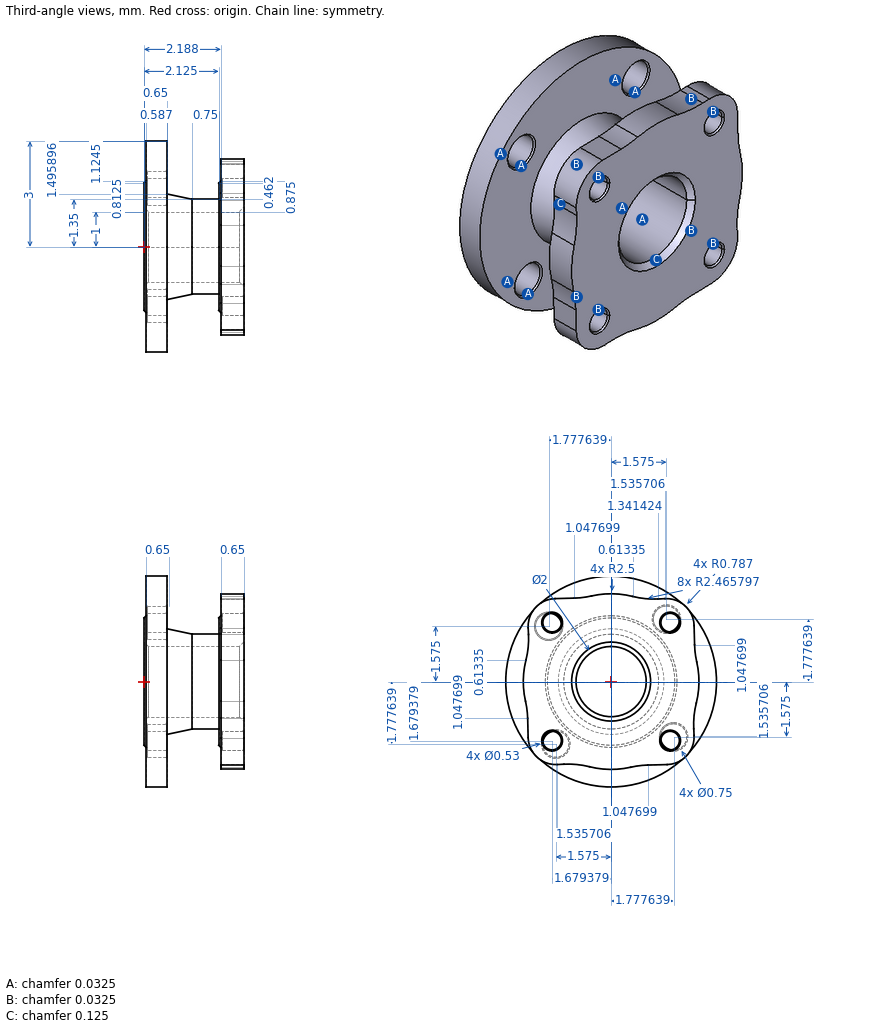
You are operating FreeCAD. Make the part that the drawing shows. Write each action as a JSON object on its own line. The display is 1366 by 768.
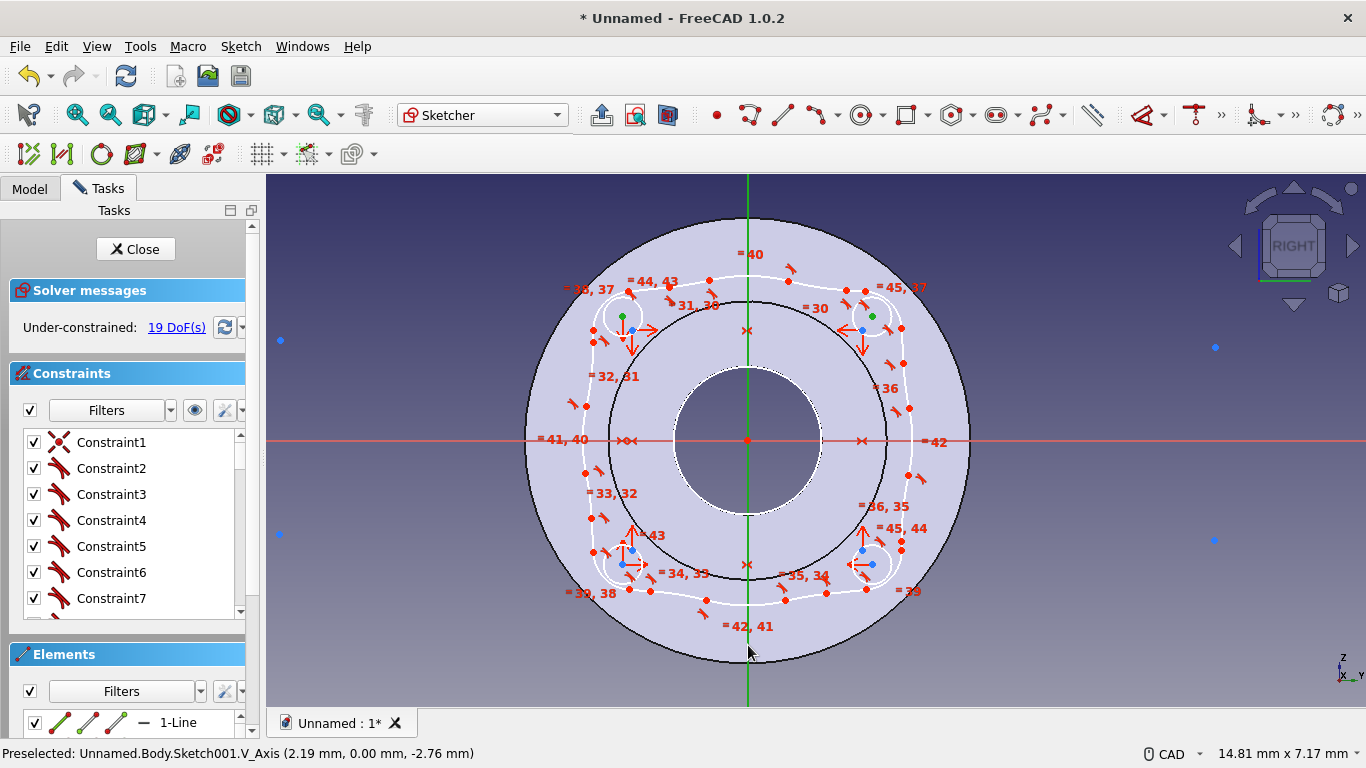
{"action": "key", "text": "s"}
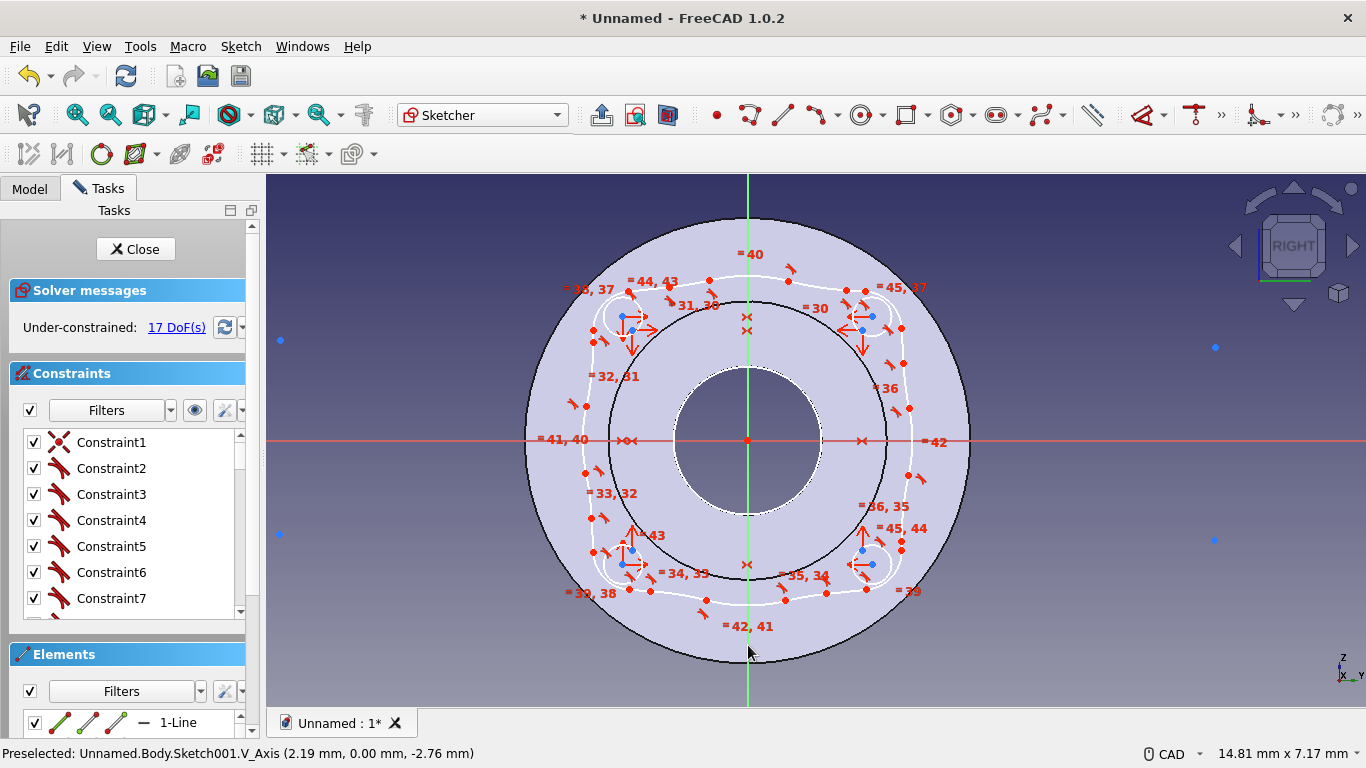
{"action": "left_click", "coordinate": [1142, 116]}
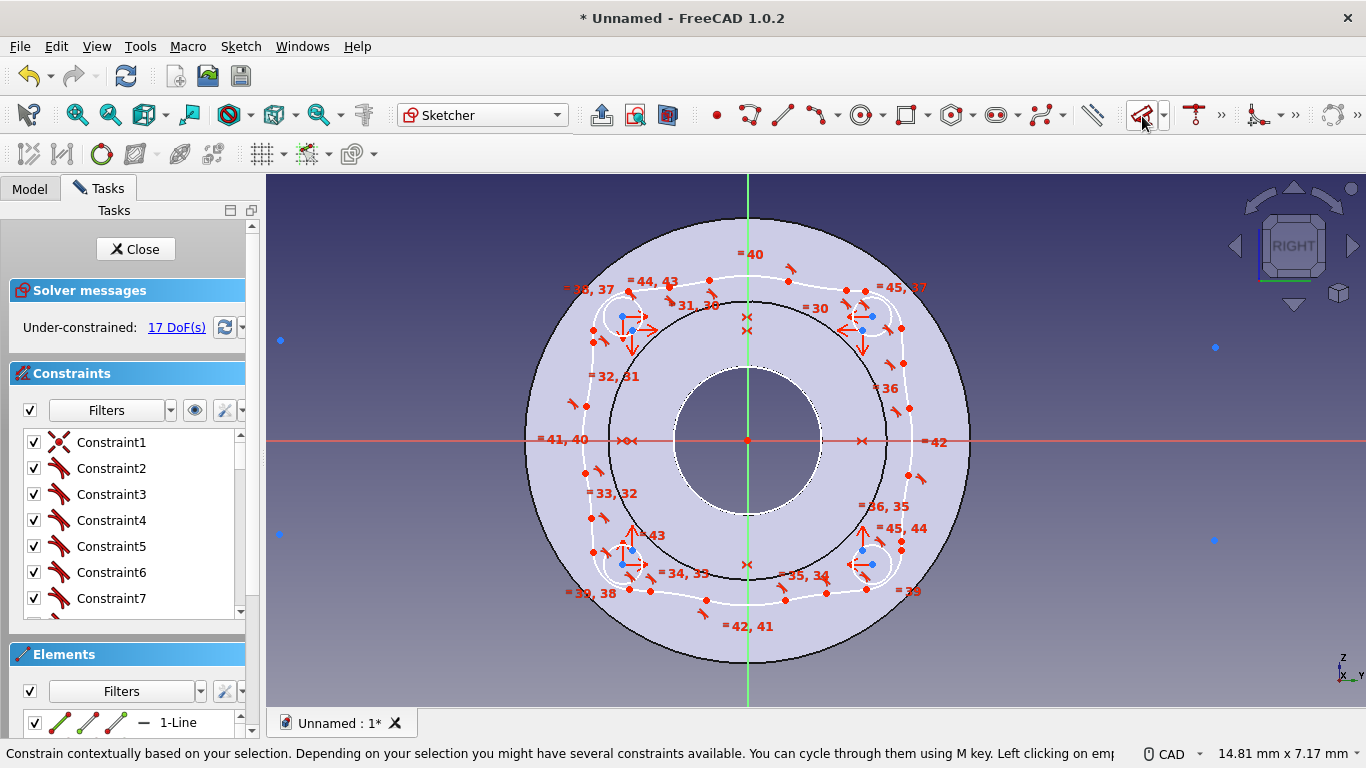
{"action": "scroll", "coordinate": [899, 317], "scroll_direction": "up", "scroll_amount": 3}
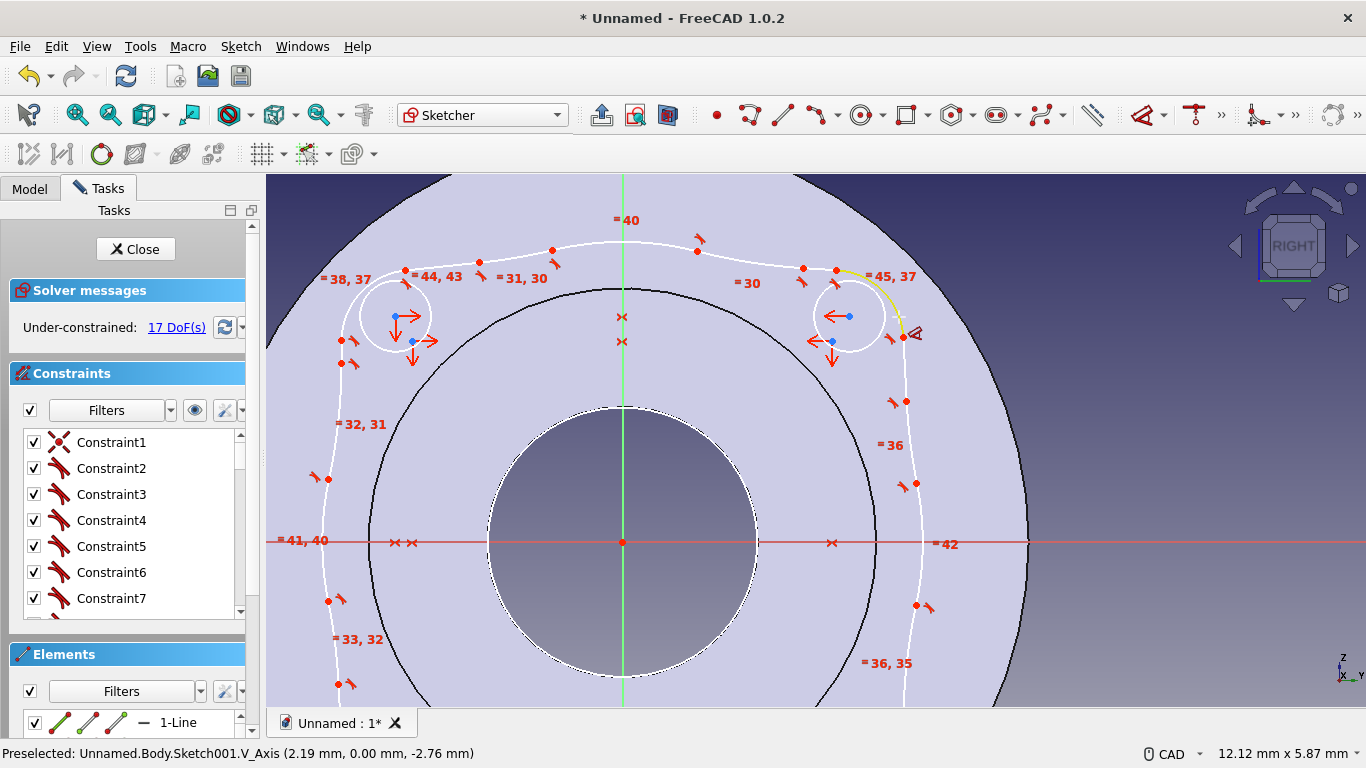
{"action": "left_click", "coordinate": [899, 317]}
{"action": "left_click", "coordinate": [929, 306]}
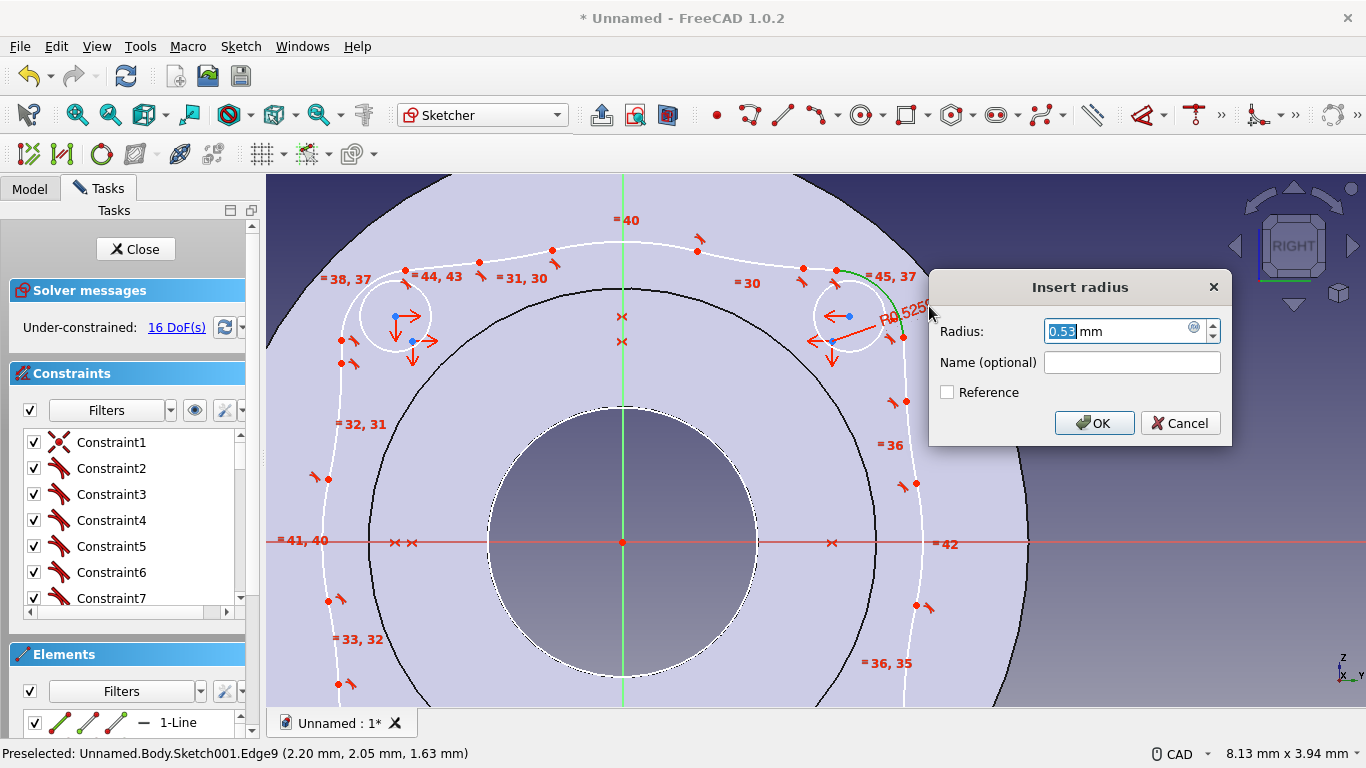
{"action": "type", "text": "0.787"}
{"action": "key", "text": "Return"}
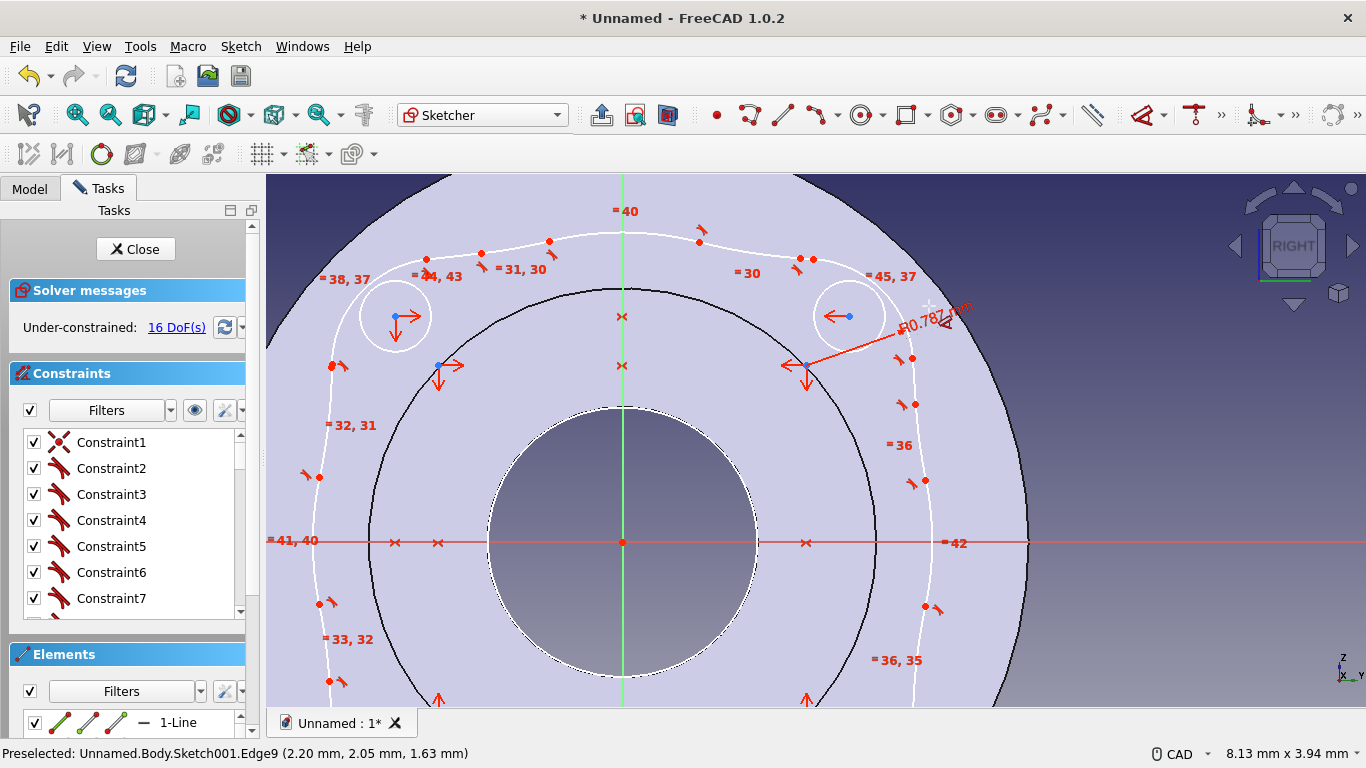
{"action": "left_click", "coordinate": [729, 249]}
{"action": "left_click", "coordinate": [723, 280]}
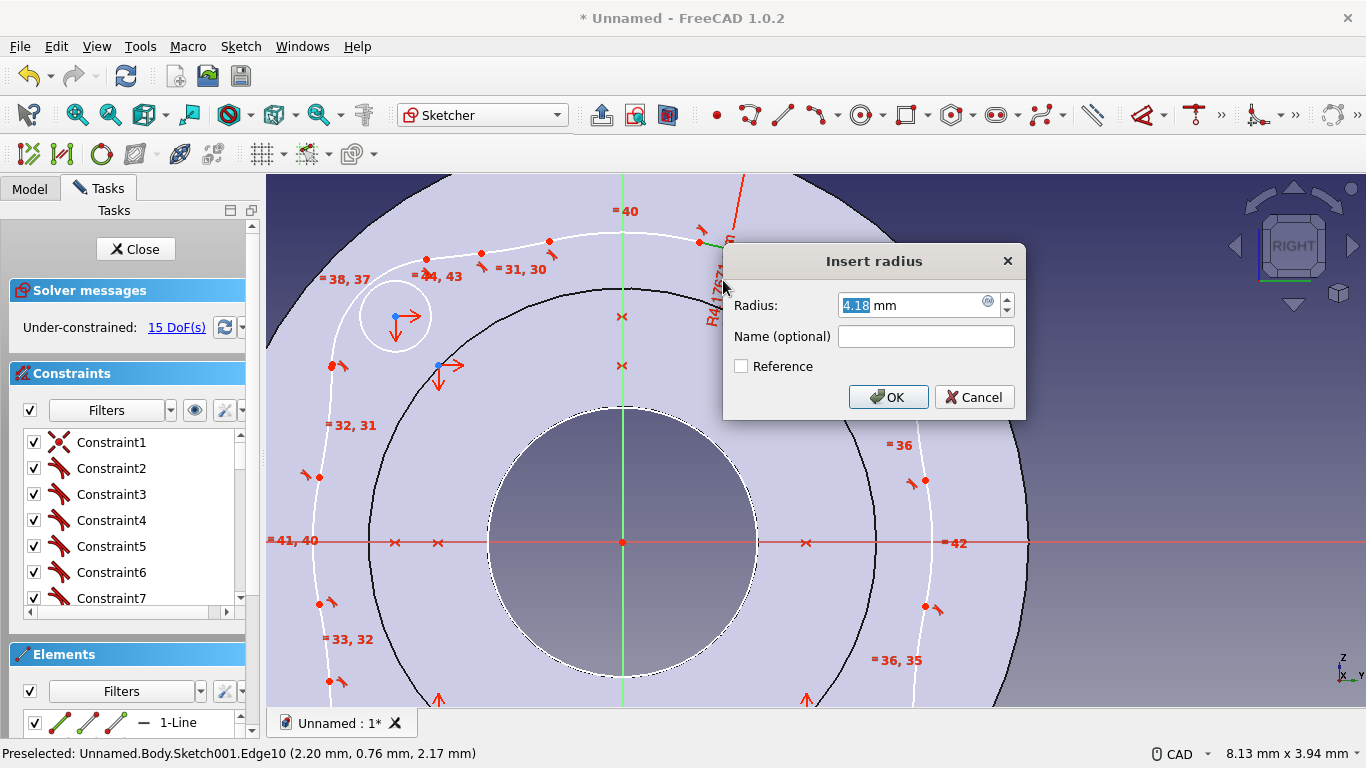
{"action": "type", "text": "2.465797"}
{"action": "key", "text": "Return"}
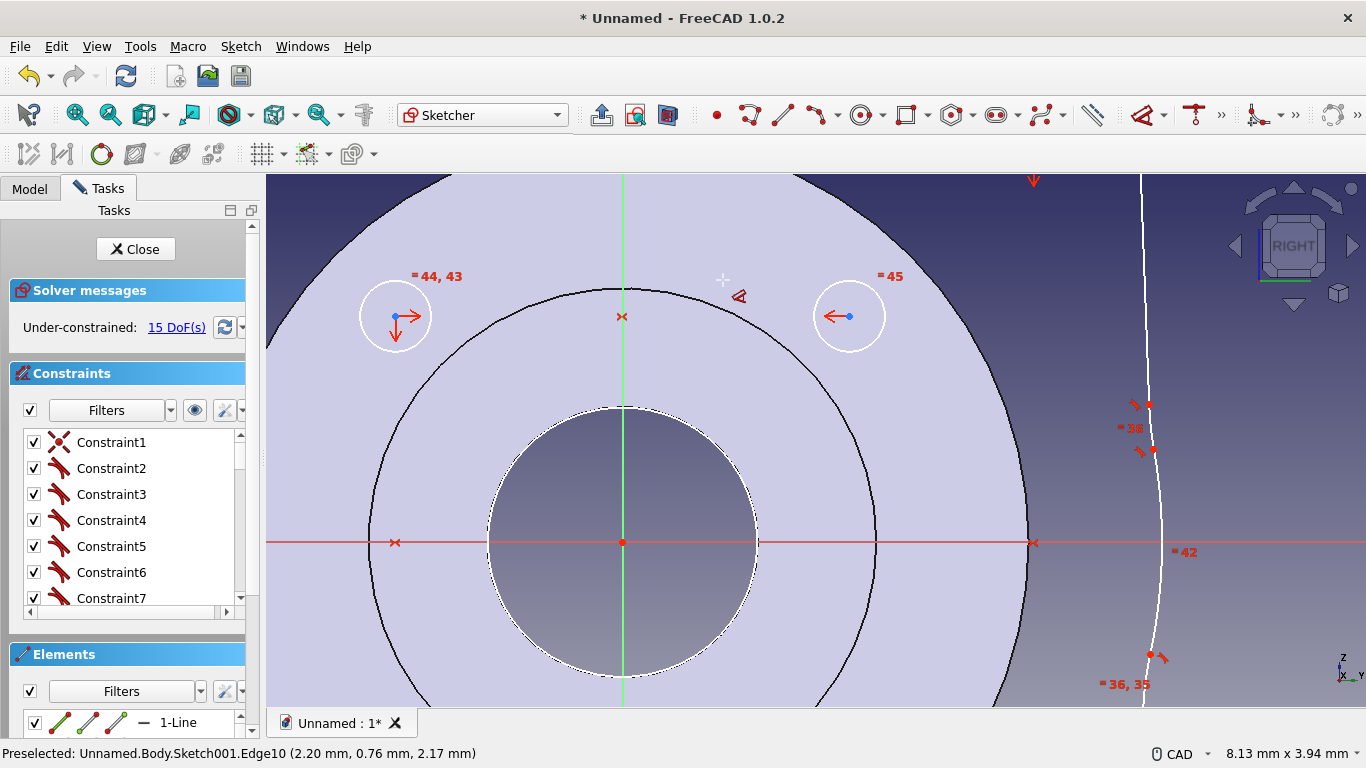
{"action": "scroll", "coordinate": [899, 317], "scroll_direction": "down", "scroll_amount": 3}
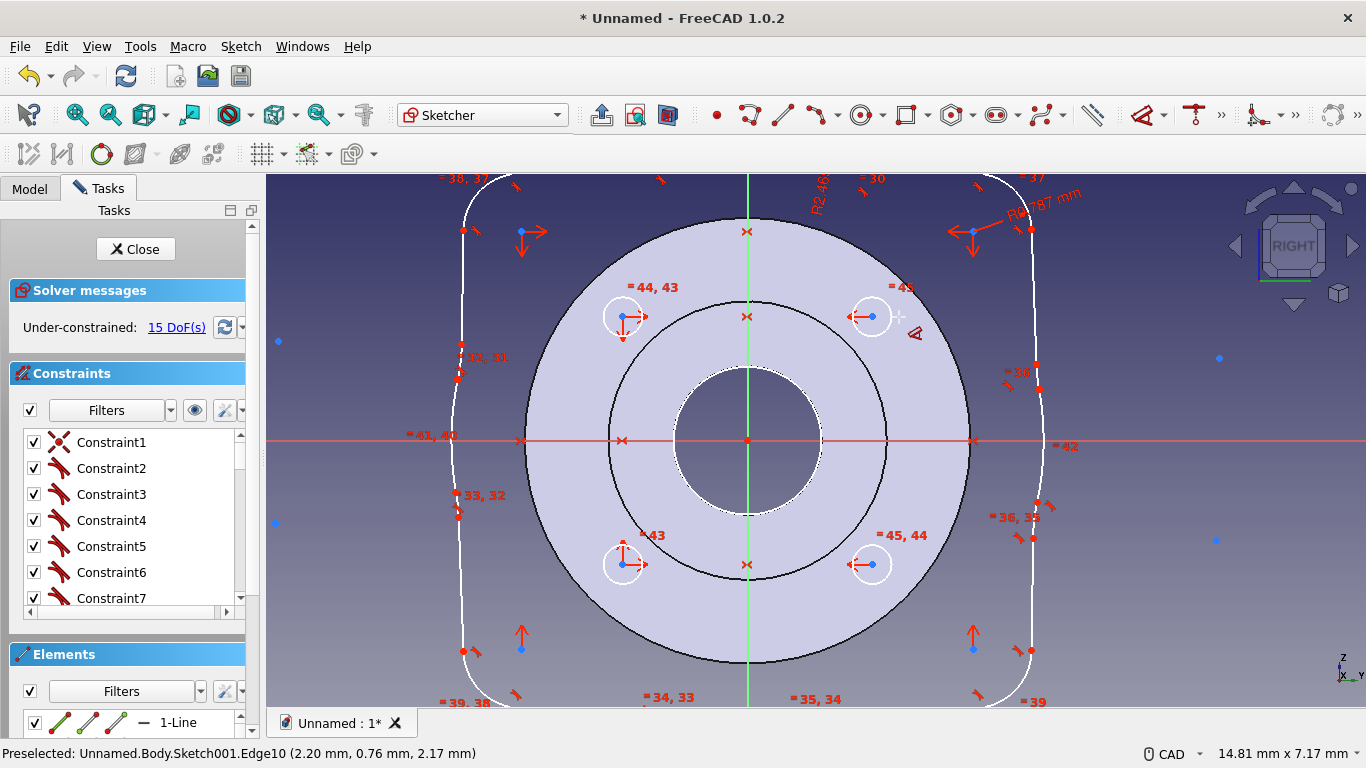
{"action": "scroll", "coordinate": [747, 550], "scroll_direction": "down", "scroll_amount": 2}